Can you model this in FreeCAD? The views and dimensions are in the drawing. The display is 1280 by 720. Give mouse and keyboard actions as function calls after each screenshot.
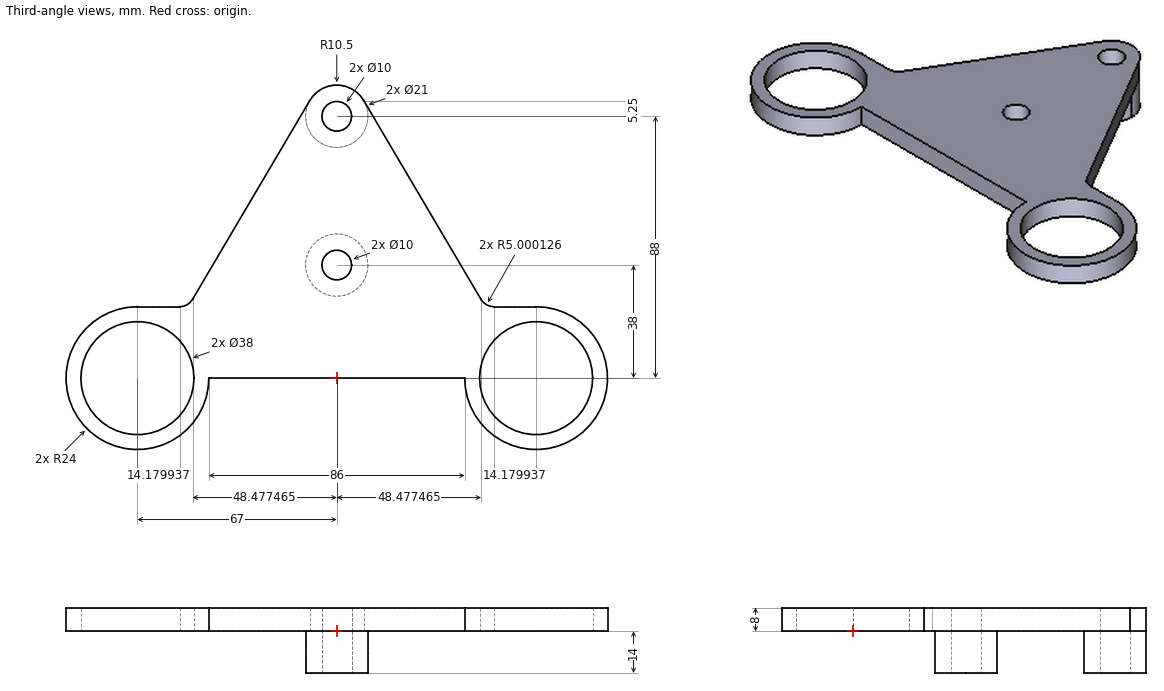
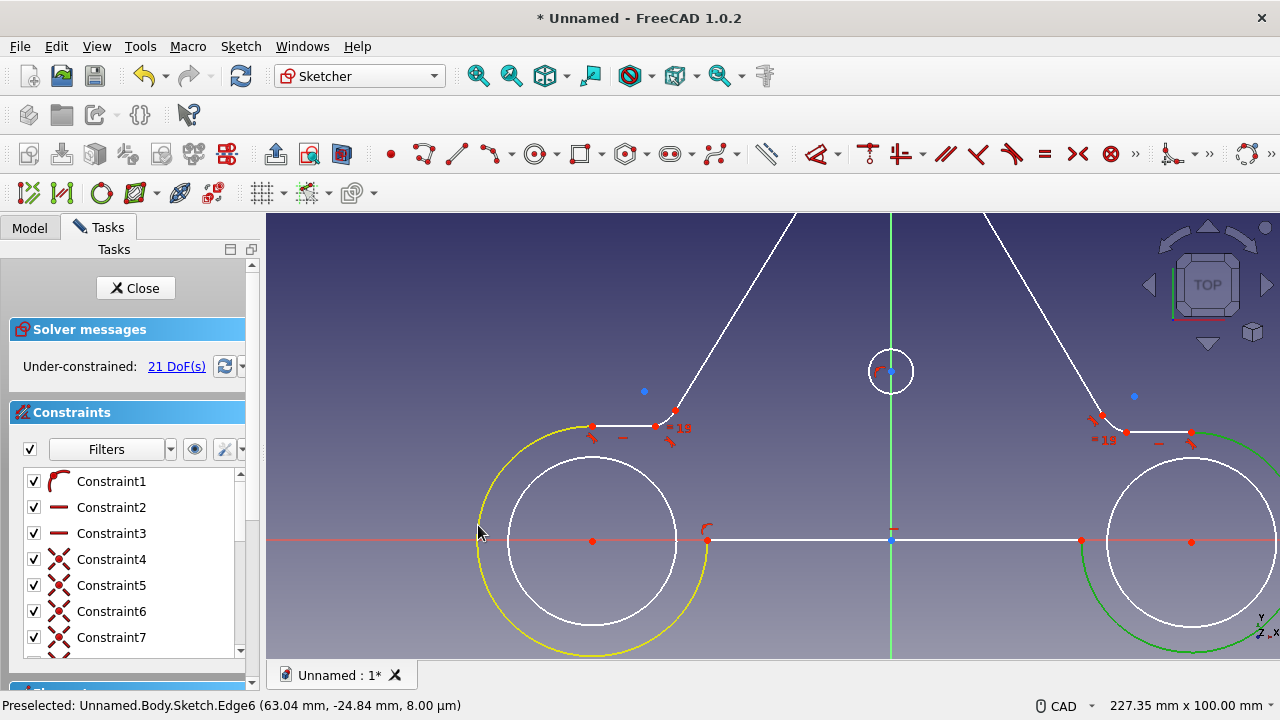
click(479, 524)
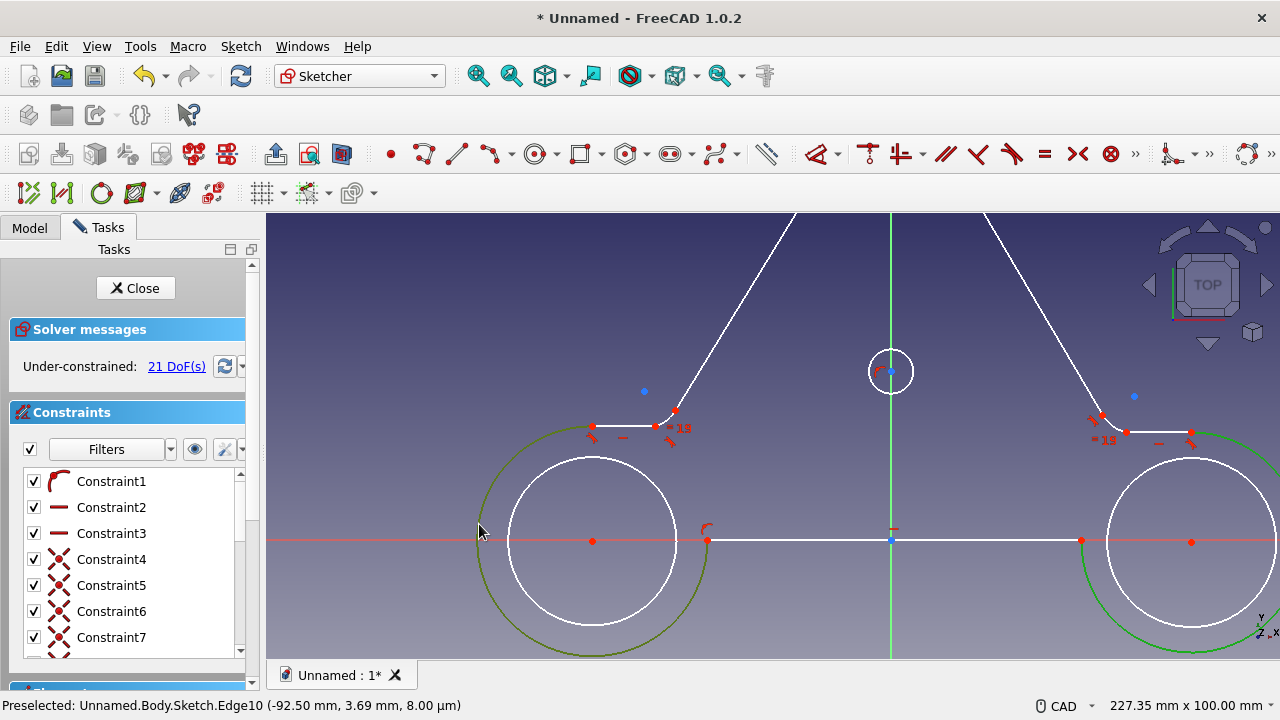
key(e)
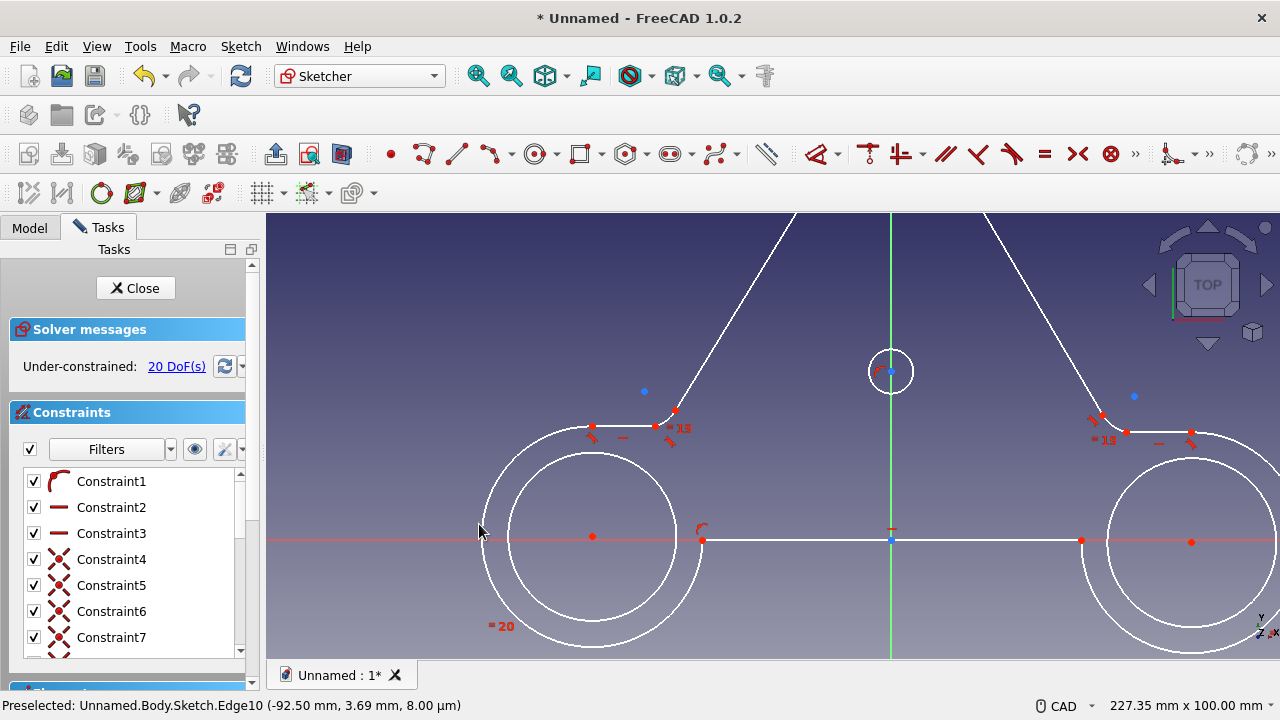
click(652, 477)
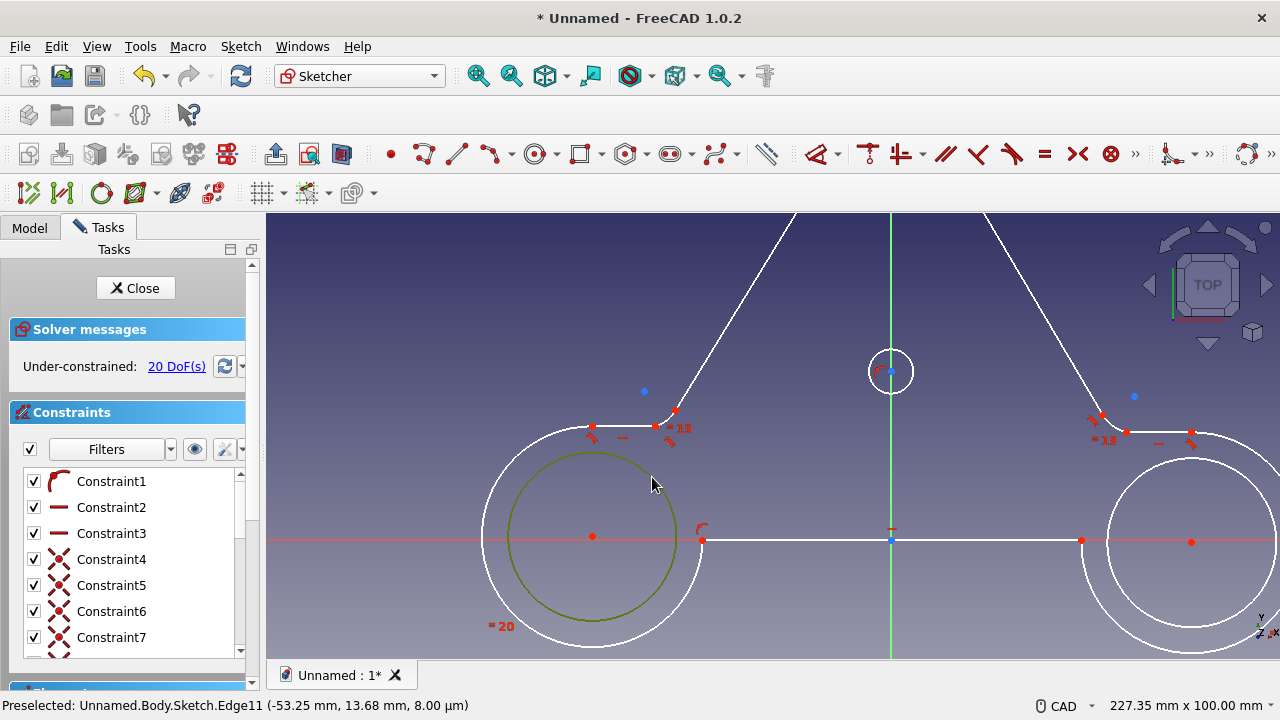
click(1107, 540)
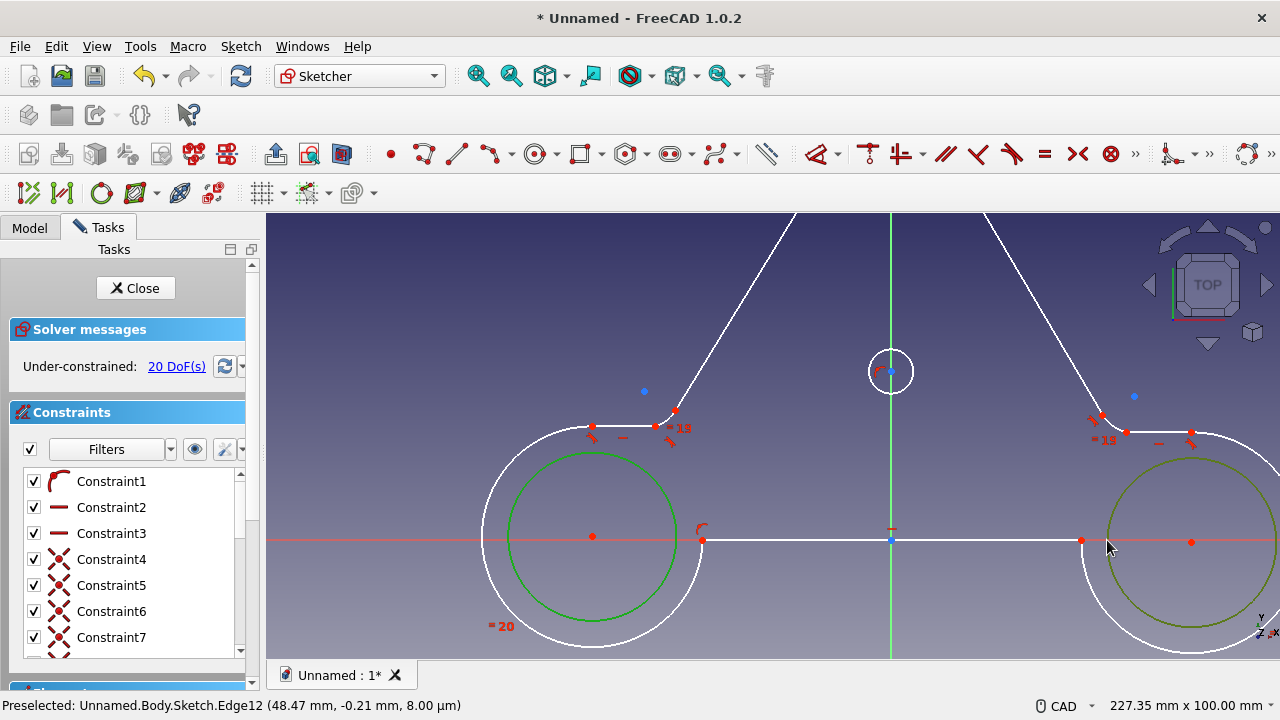
key(e)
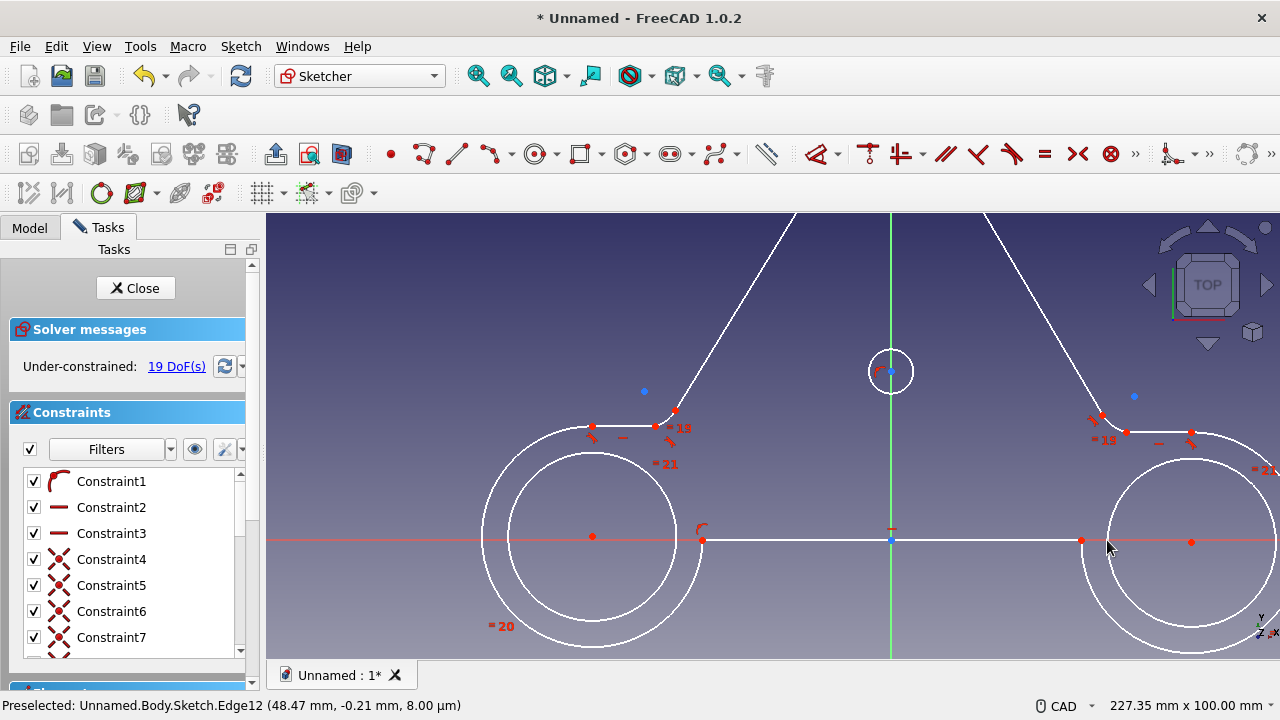
click(907, 356)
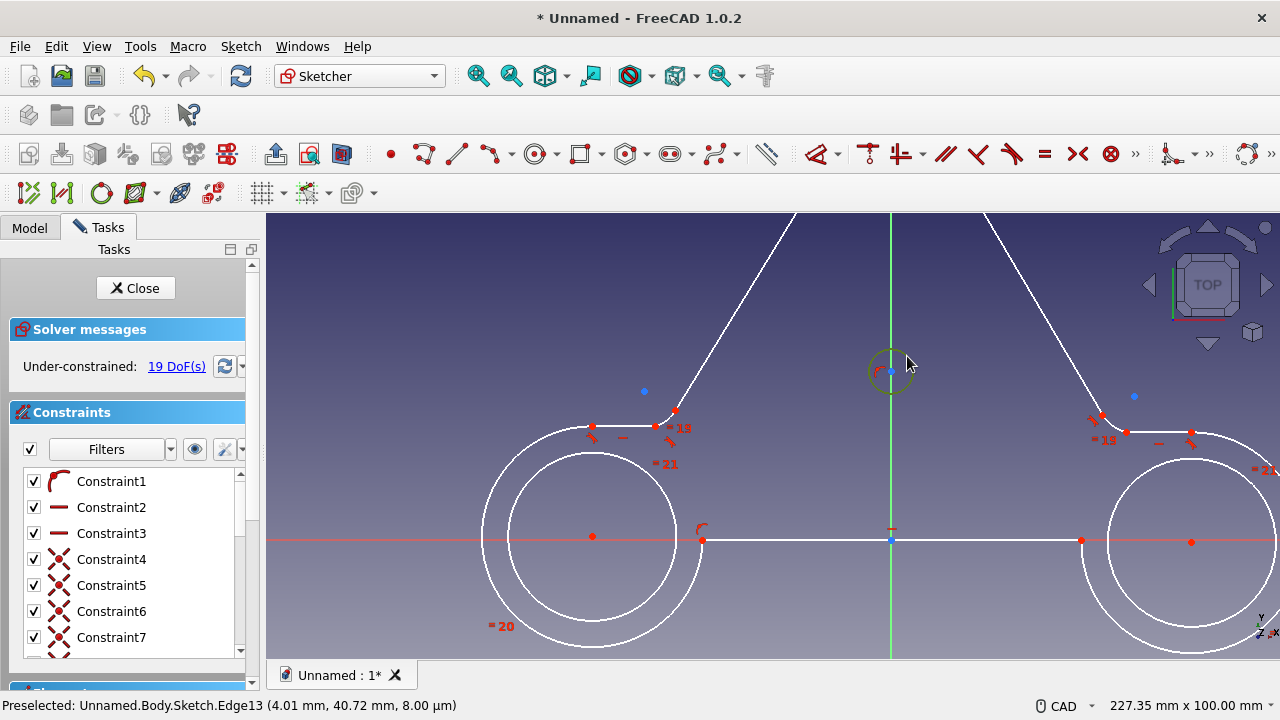
scroll(477, 525, down, 3)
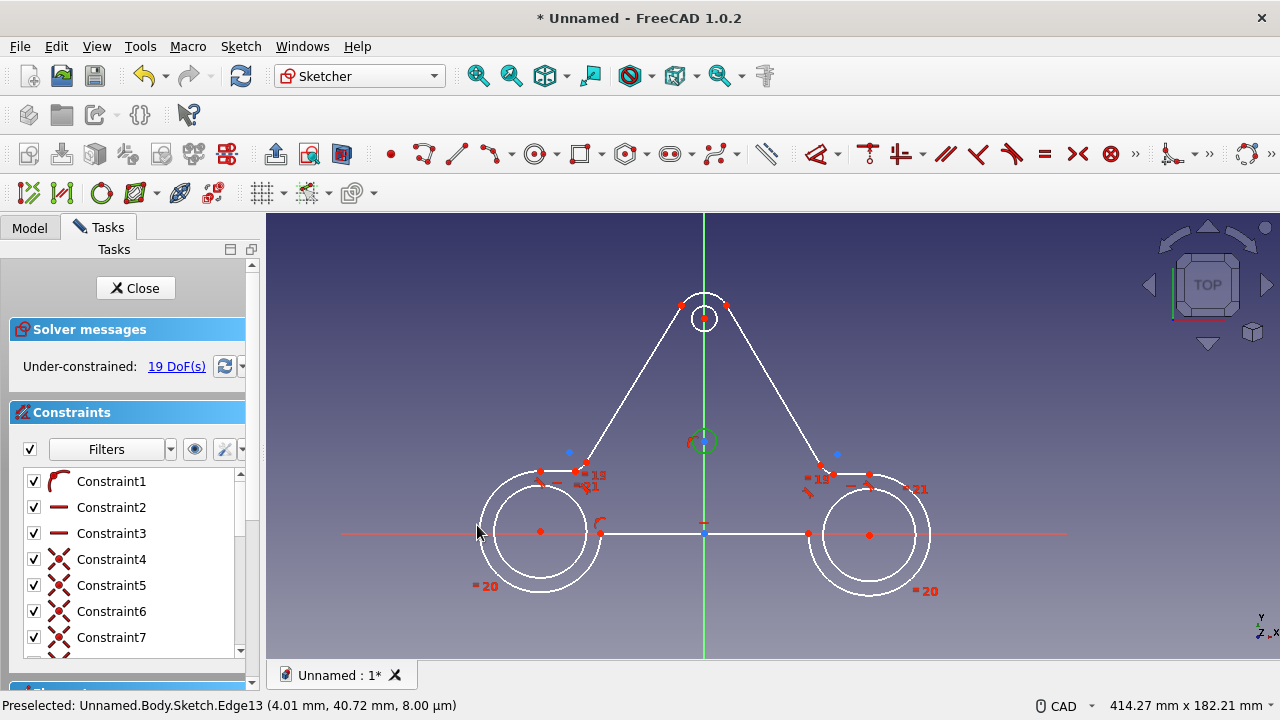
scroll(713, 310, up, 3)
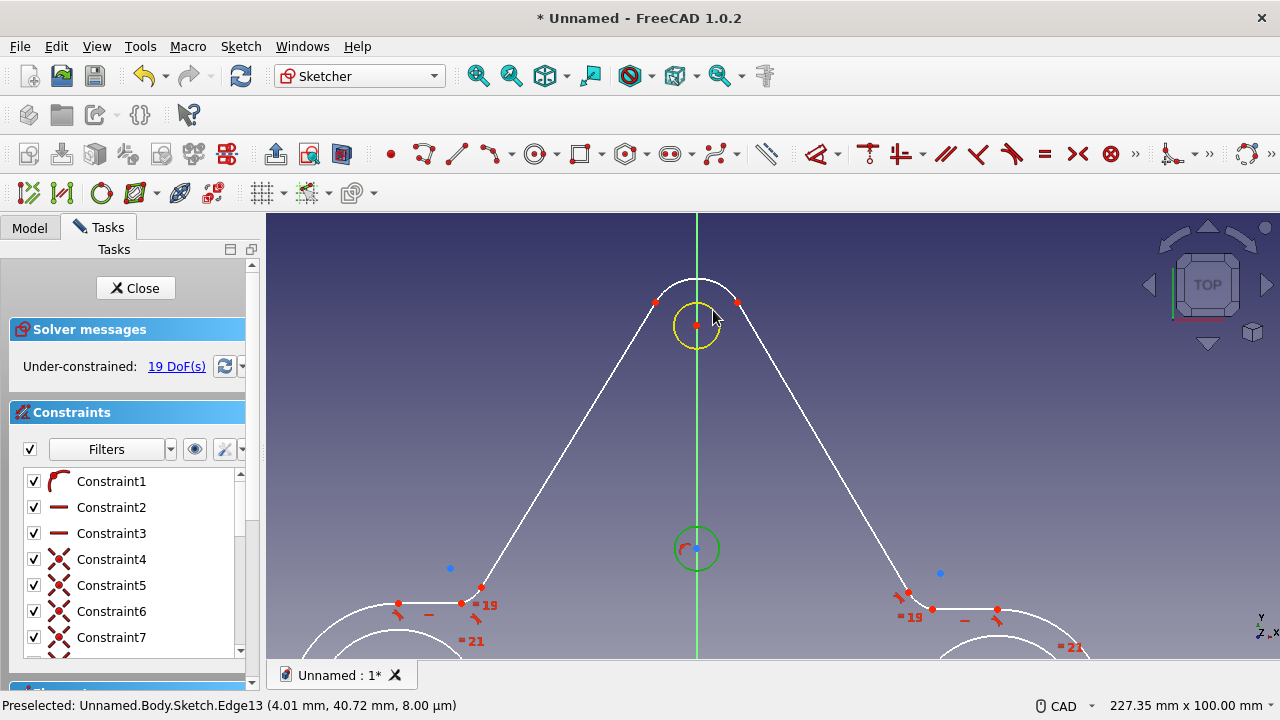
click(713, 310)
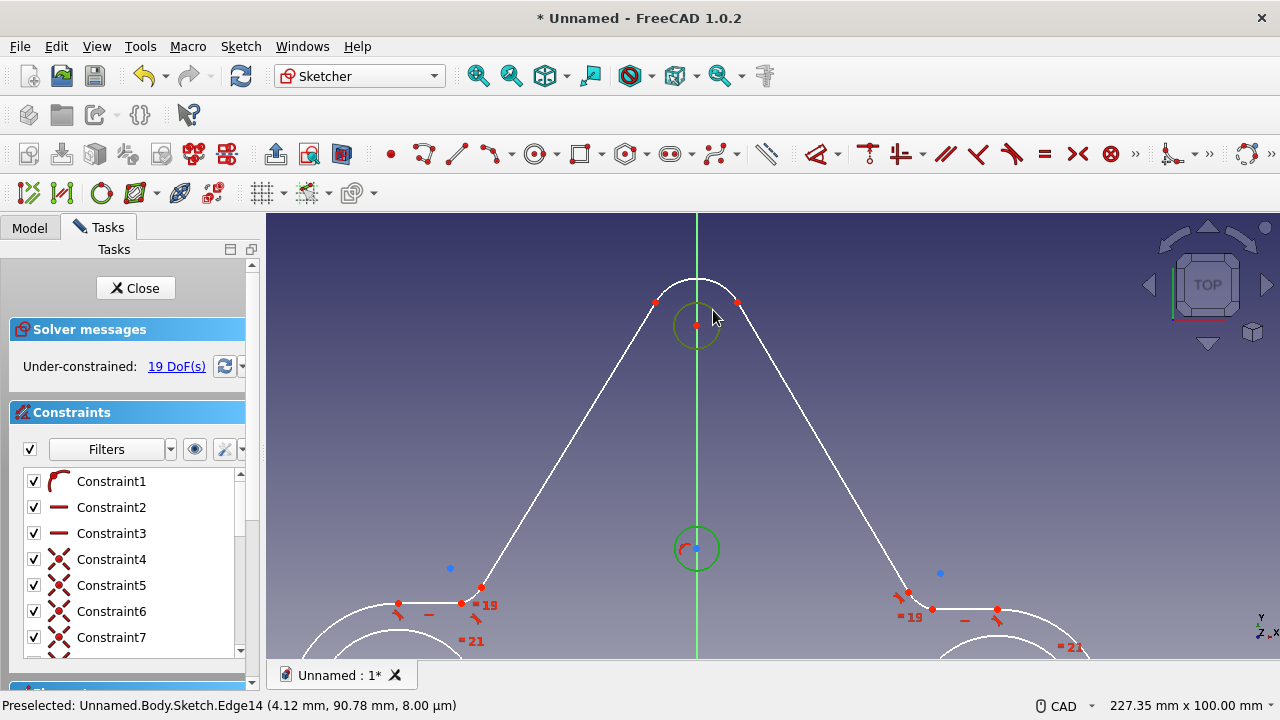
key(e)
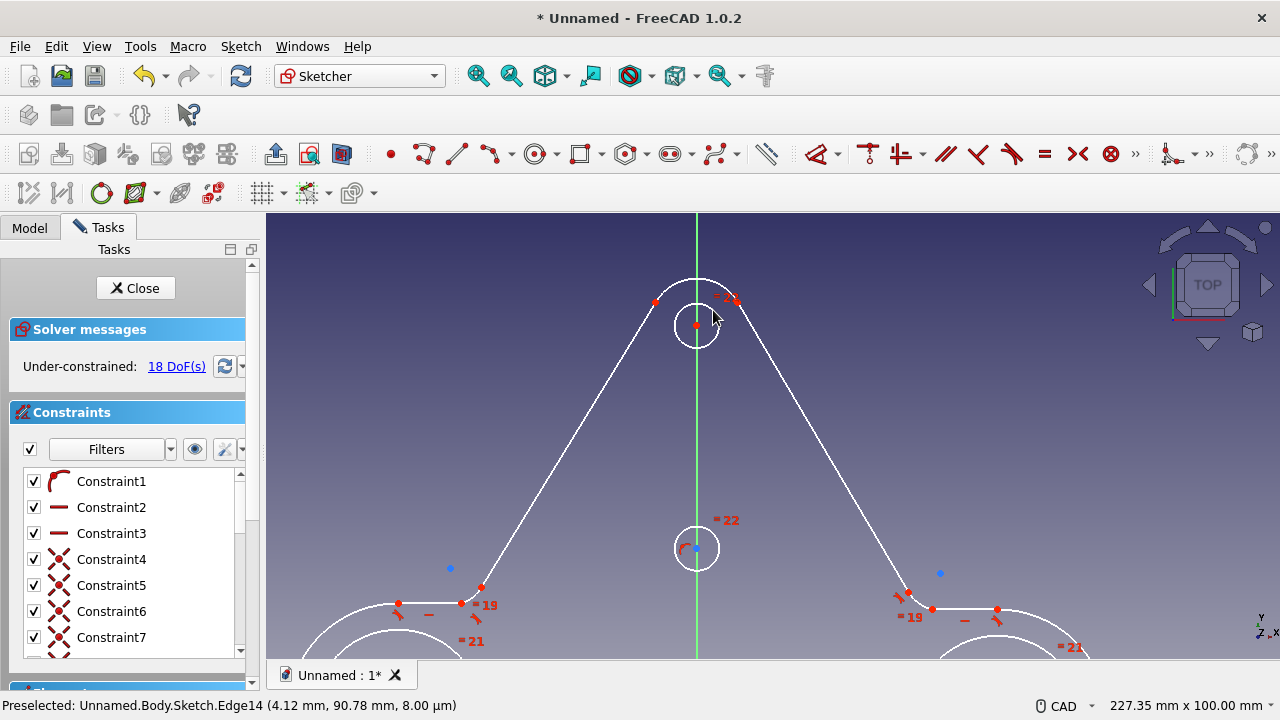
scroll(714, 310, down, 3)